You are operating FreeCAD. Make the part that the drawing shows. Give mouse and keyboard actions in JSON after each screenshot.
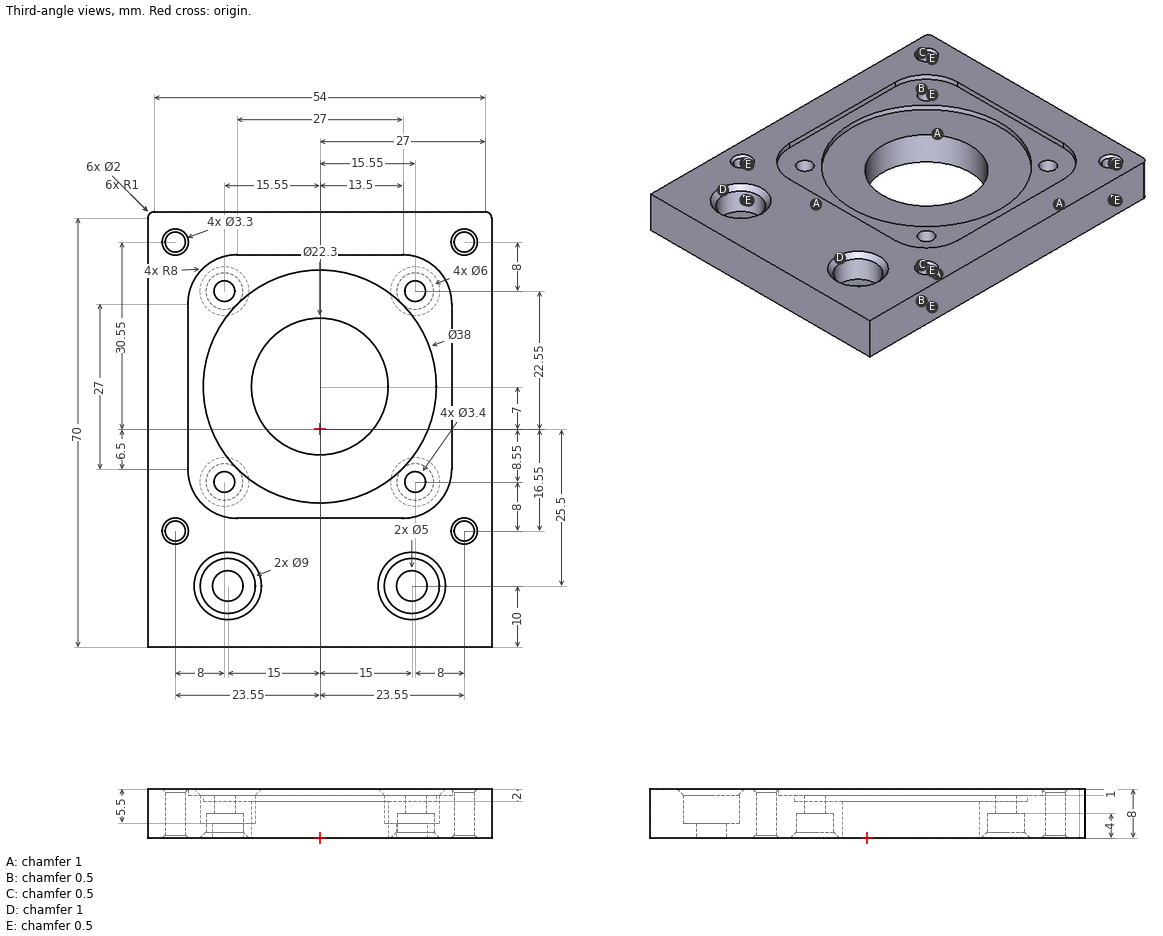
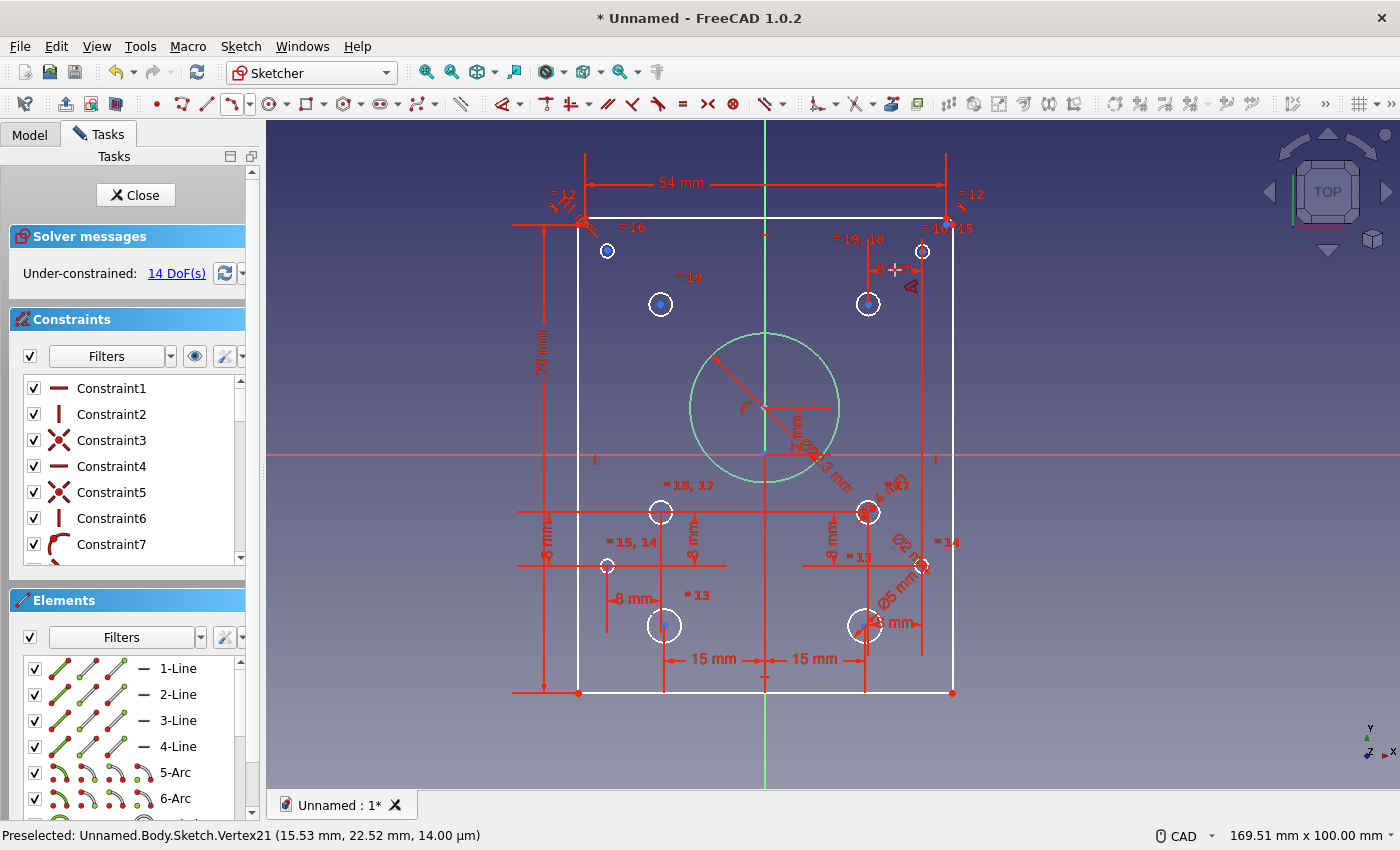
{"action": "left_click", "coordinate": [868, 304]}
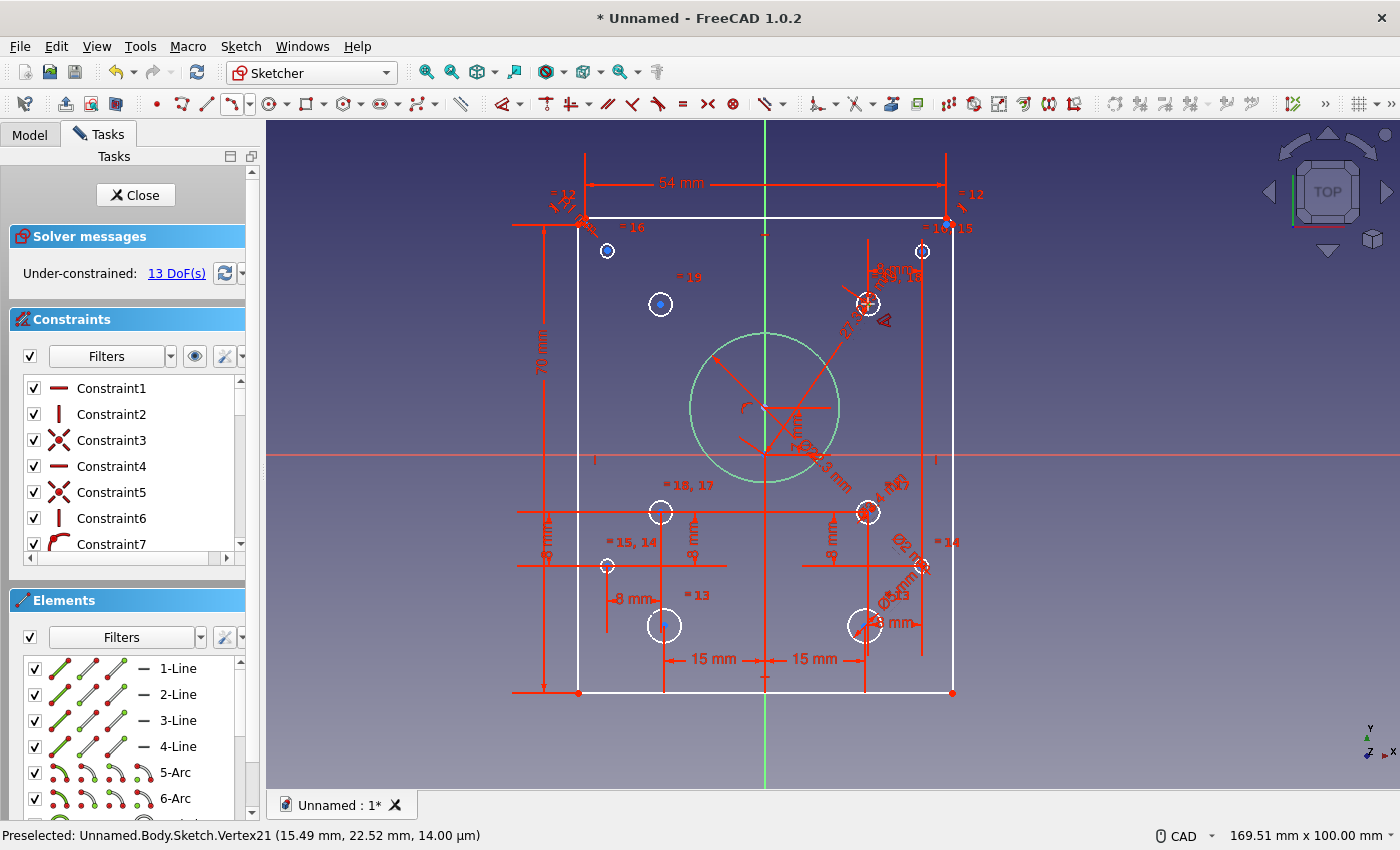
{"action": "left_click", "coordinate": [923, 252]}
{"action": "left_click", "coordinate": [895, 338]}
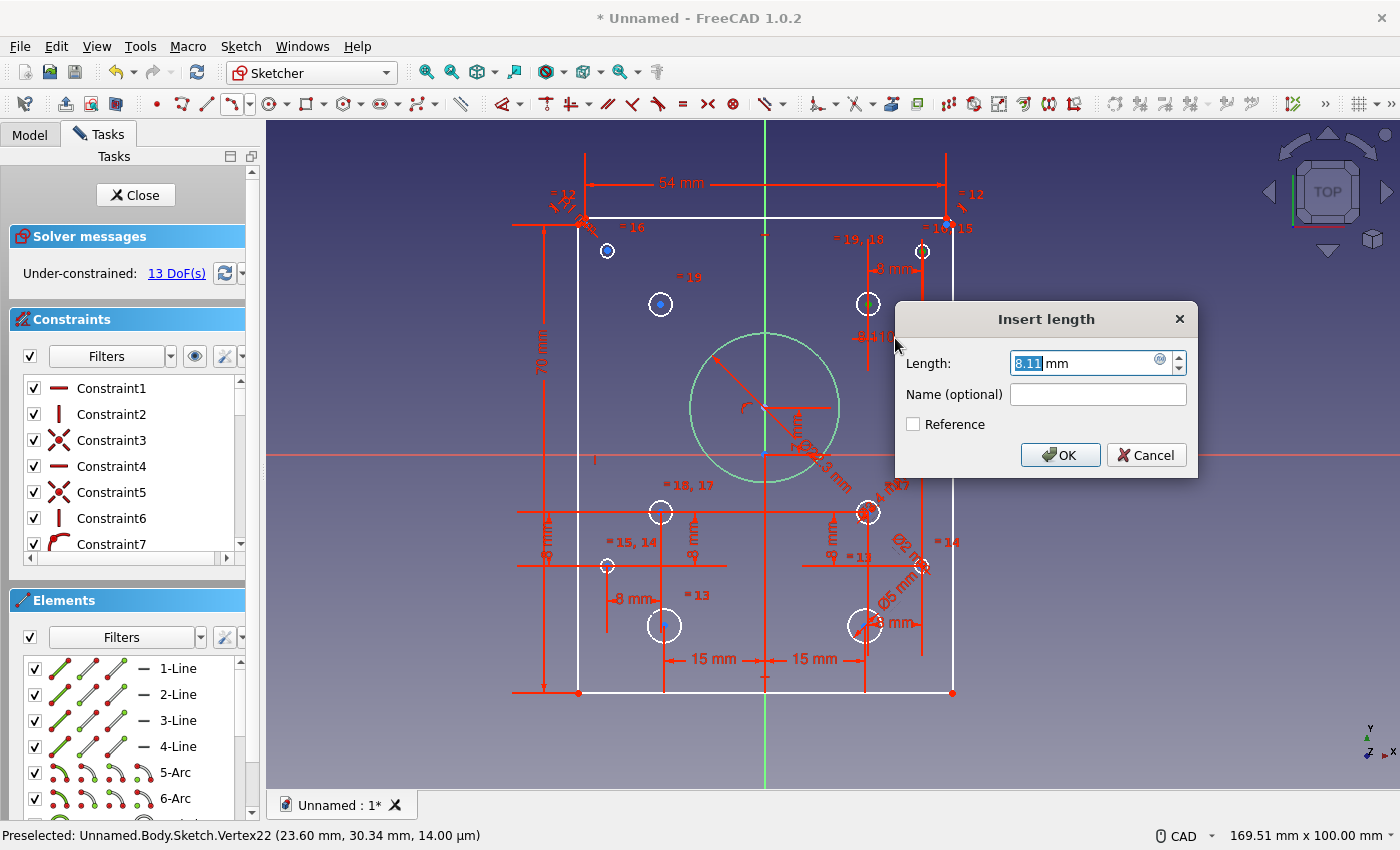
{"action": "type", "text": "8"}
{"action": "key", "text": "Return"}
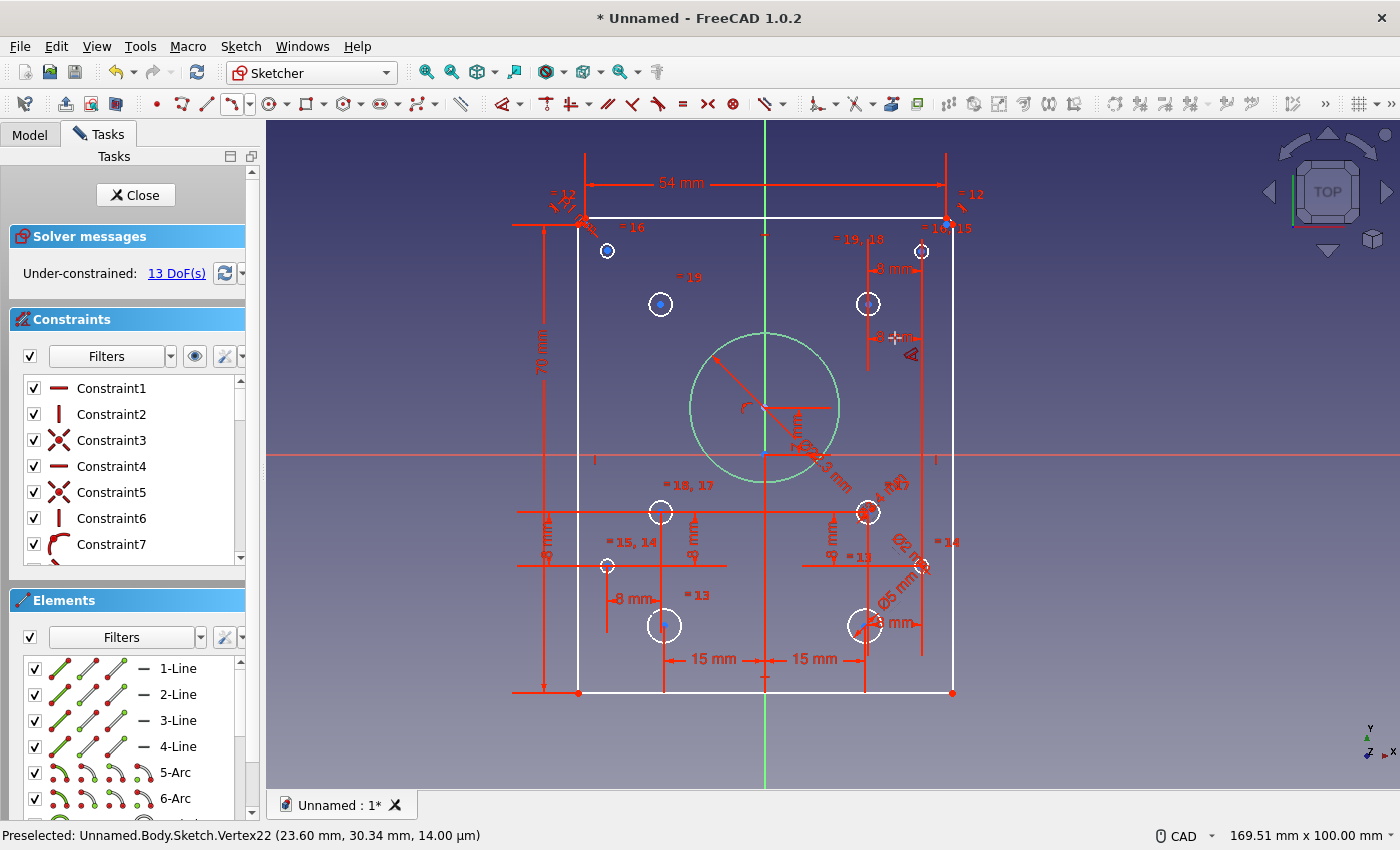
{"action": "left_click", "coordinate": [868, 304]}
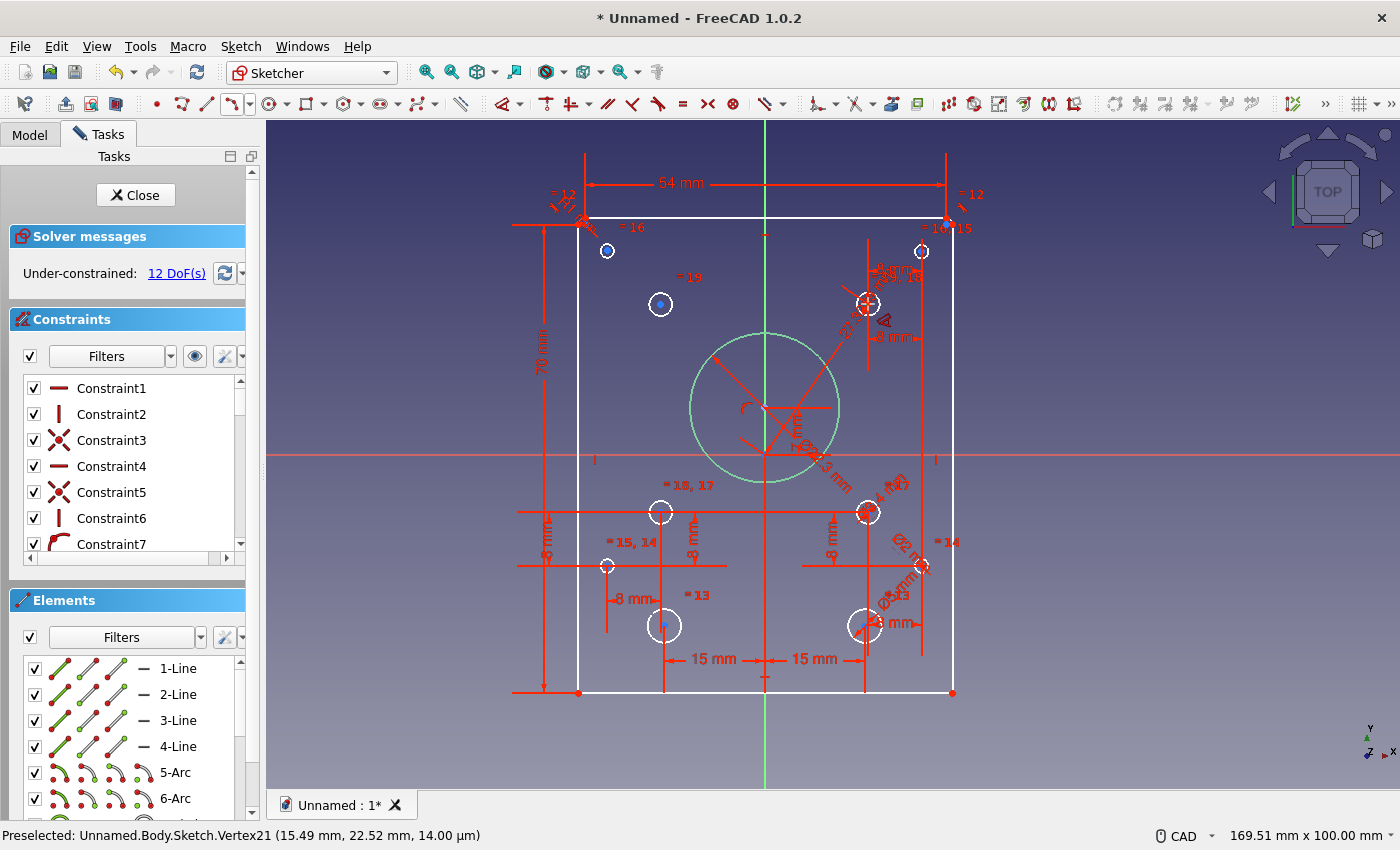
{"action": "left_click", "coordinate": [922, 252]}
{"action": "left_click", "coordinate": [834, 296]}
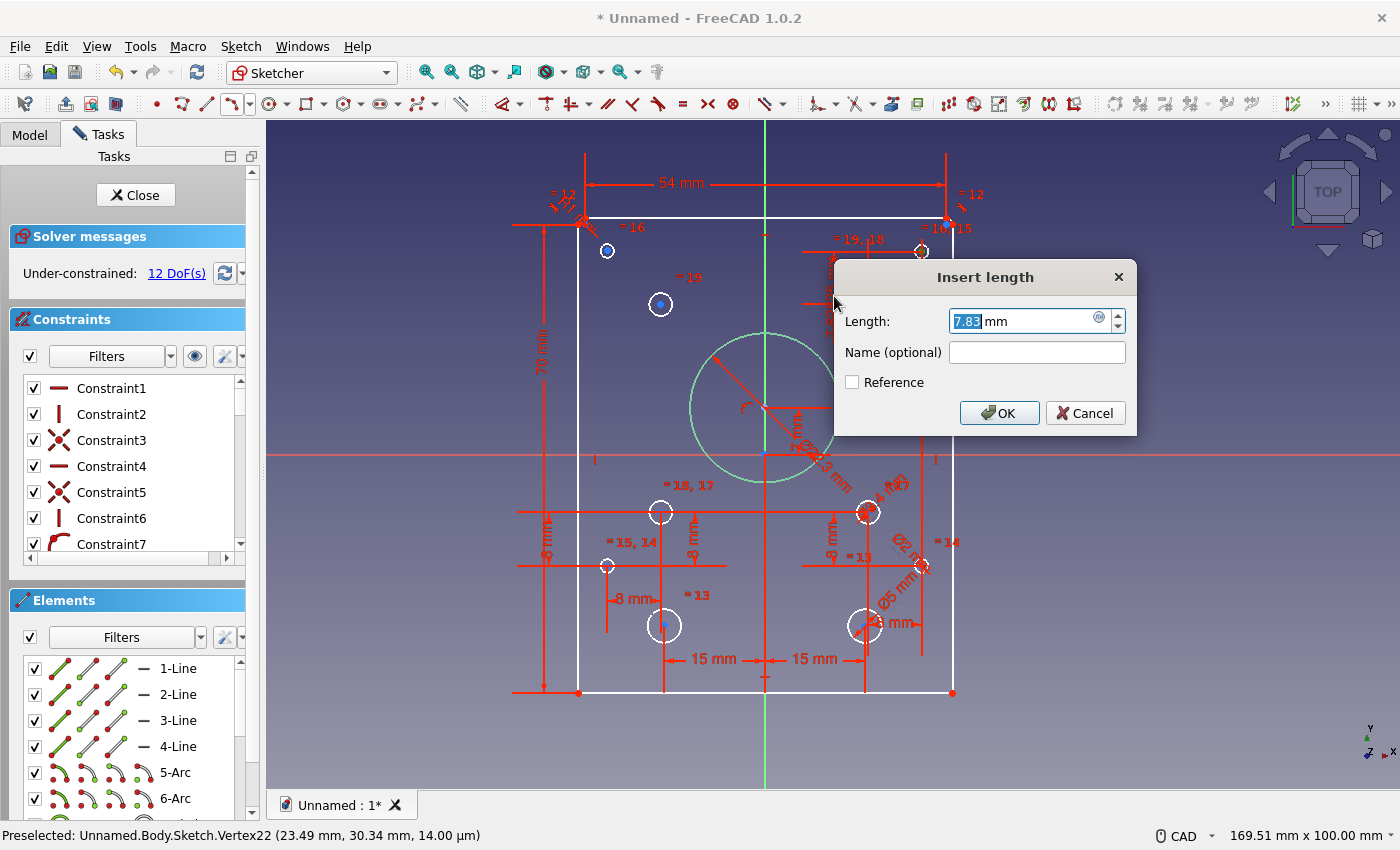
{"action": "type", "text": "8"}
{"action": "key", "text": "Return"}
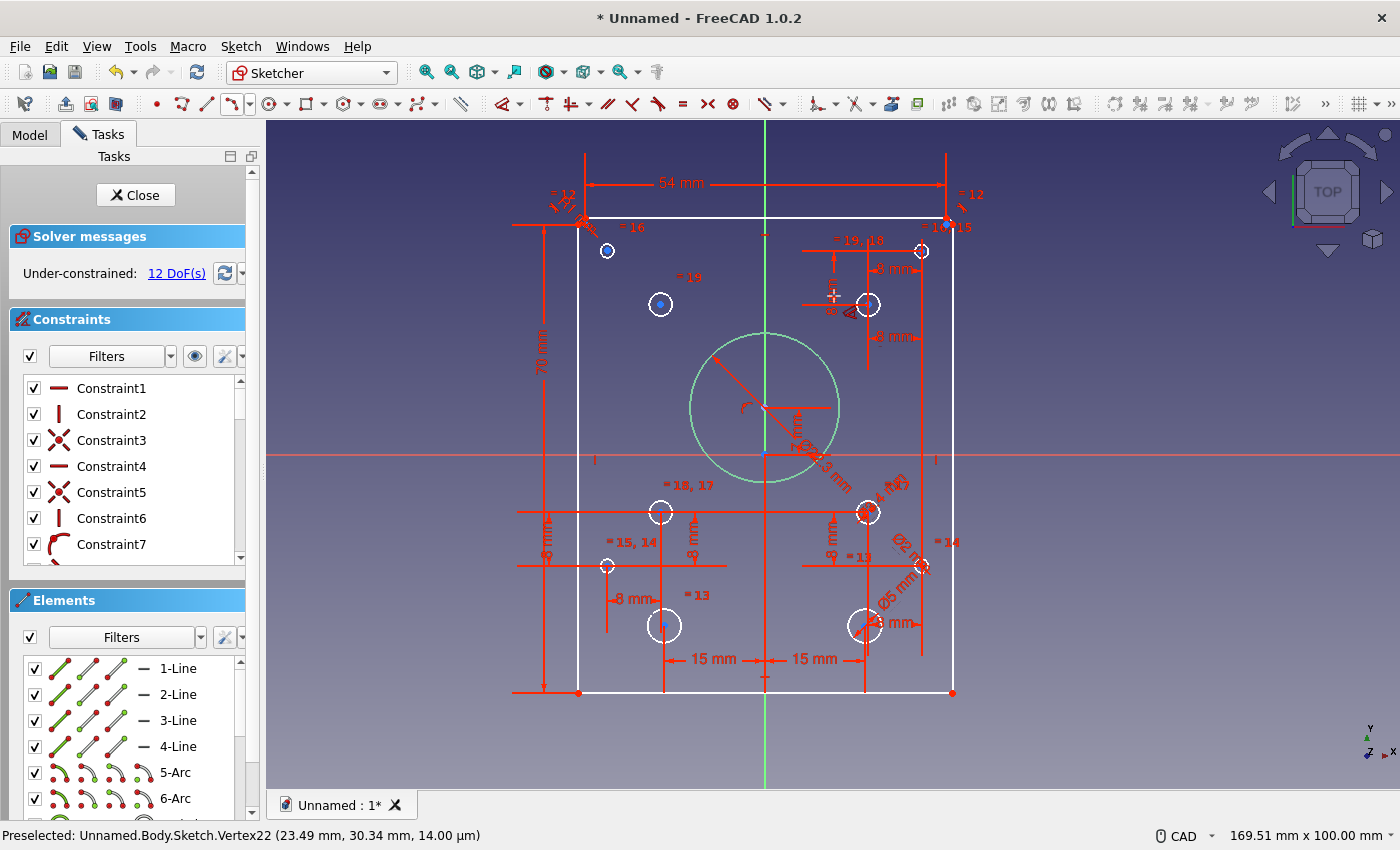
{"action": "left_click", "coordinate": [661, 305]}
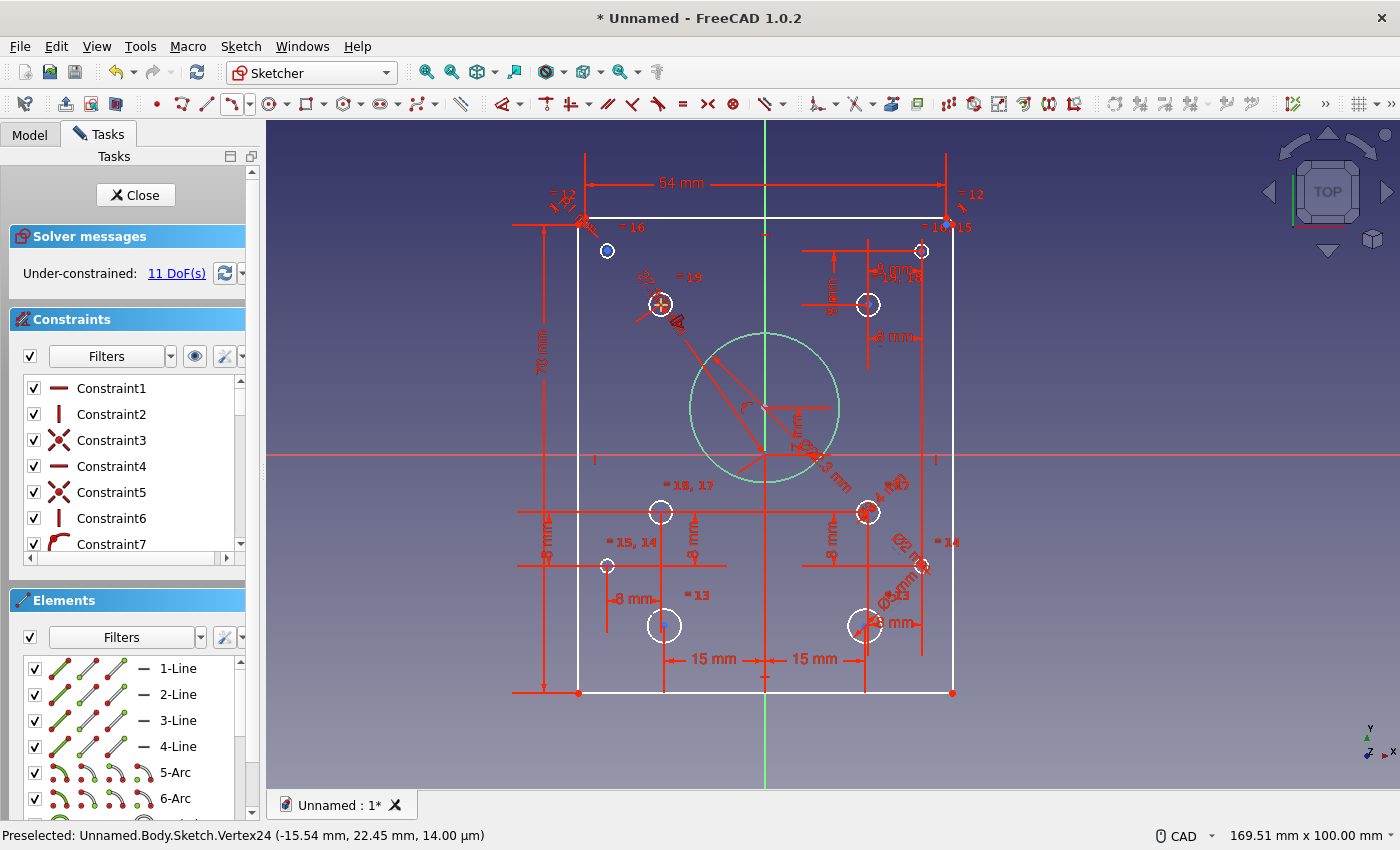
{"action": "left_click", "coordinate": [607, 251]}
{"action": "left_click", "coordinate": [634, 339]}